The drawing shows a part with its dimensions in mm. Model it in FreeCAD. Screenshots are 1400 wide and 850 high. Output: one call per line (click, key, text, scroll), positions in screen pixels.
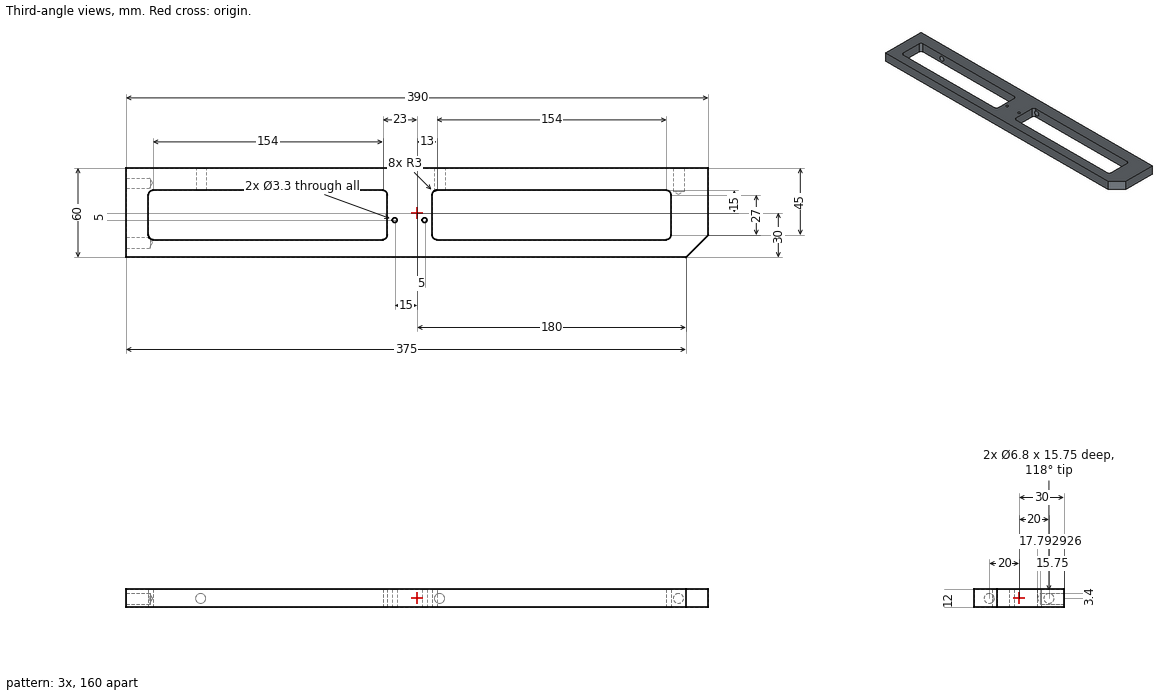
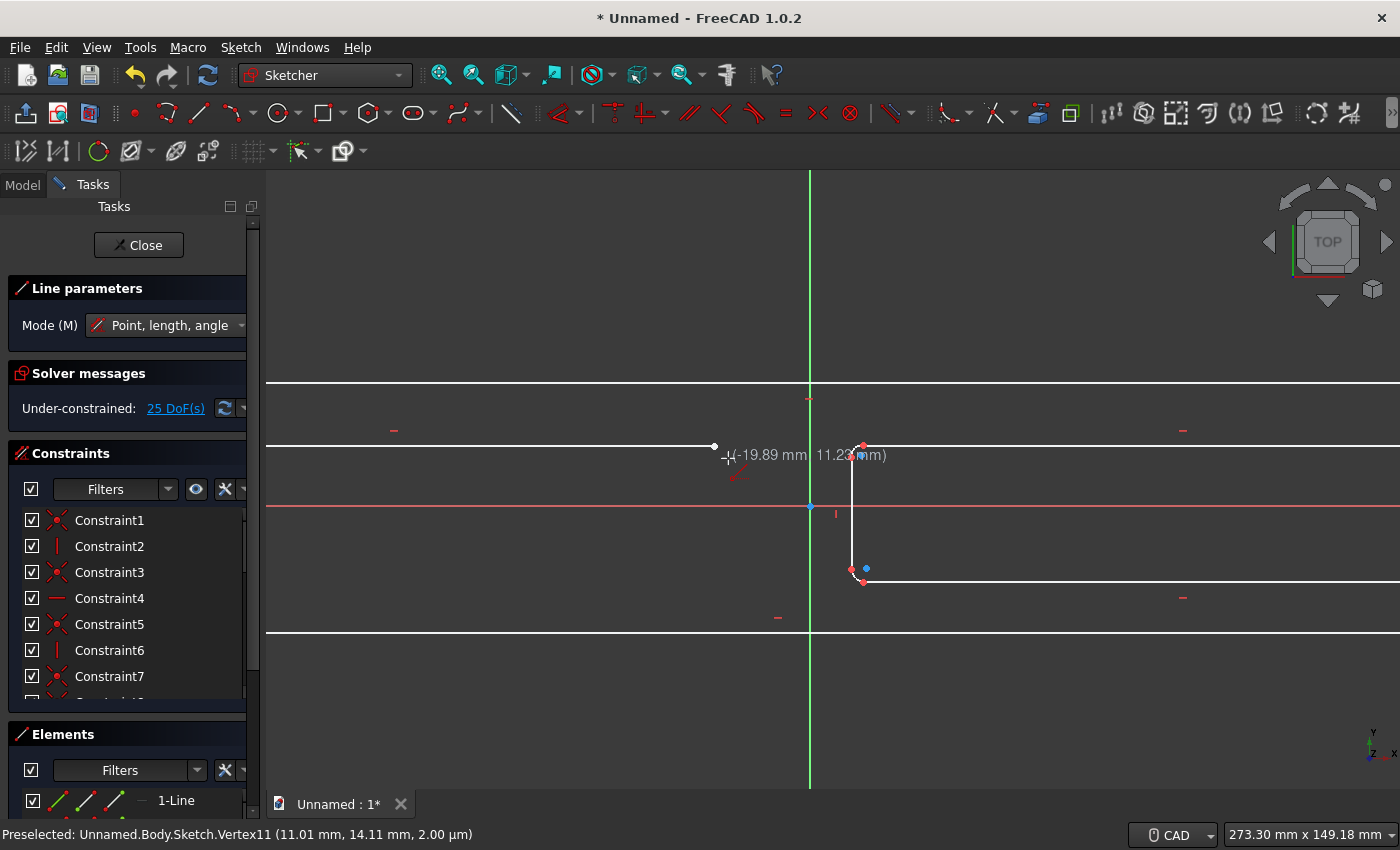
click(727, 456)
click(727, 568)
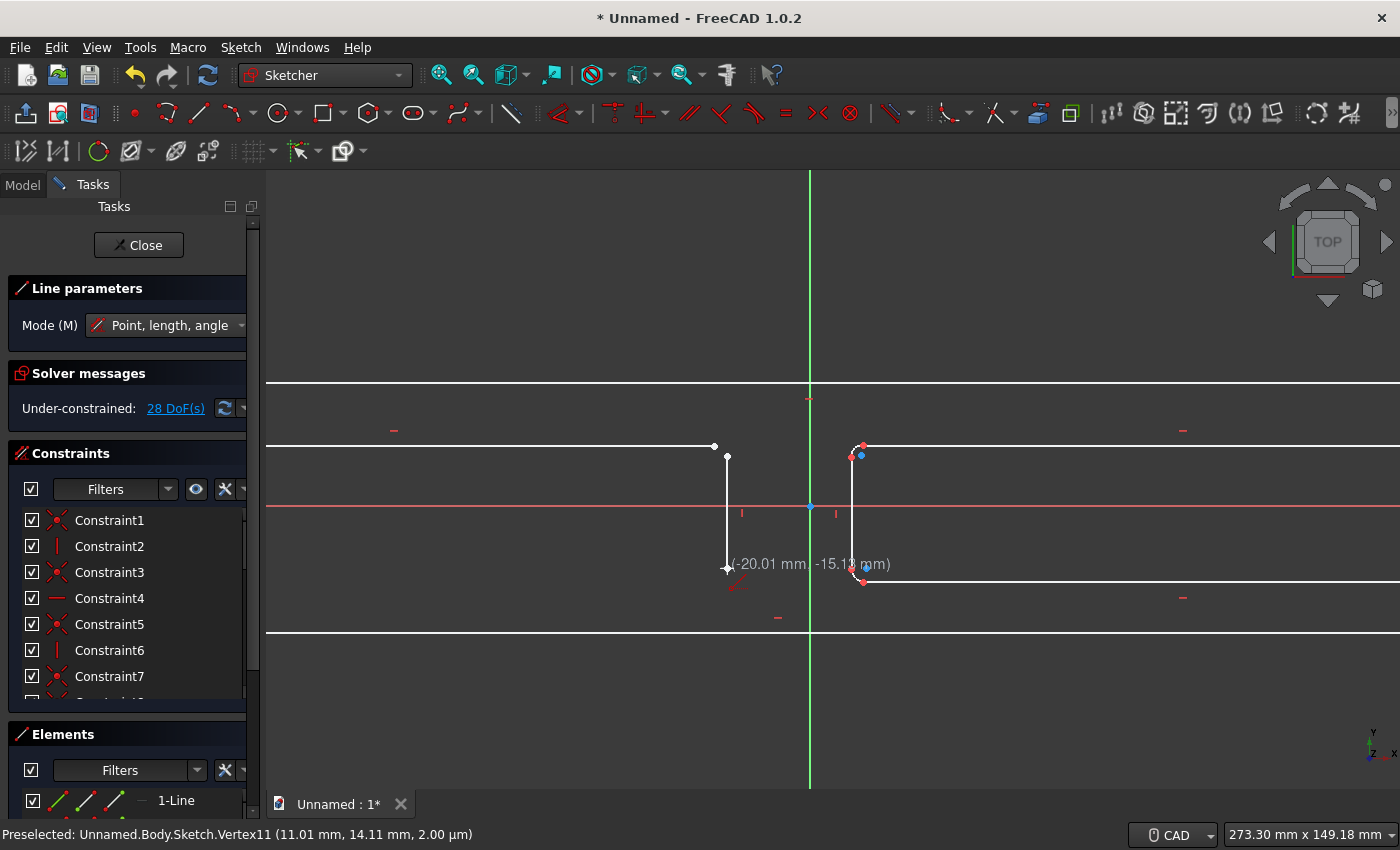
click(715, 581)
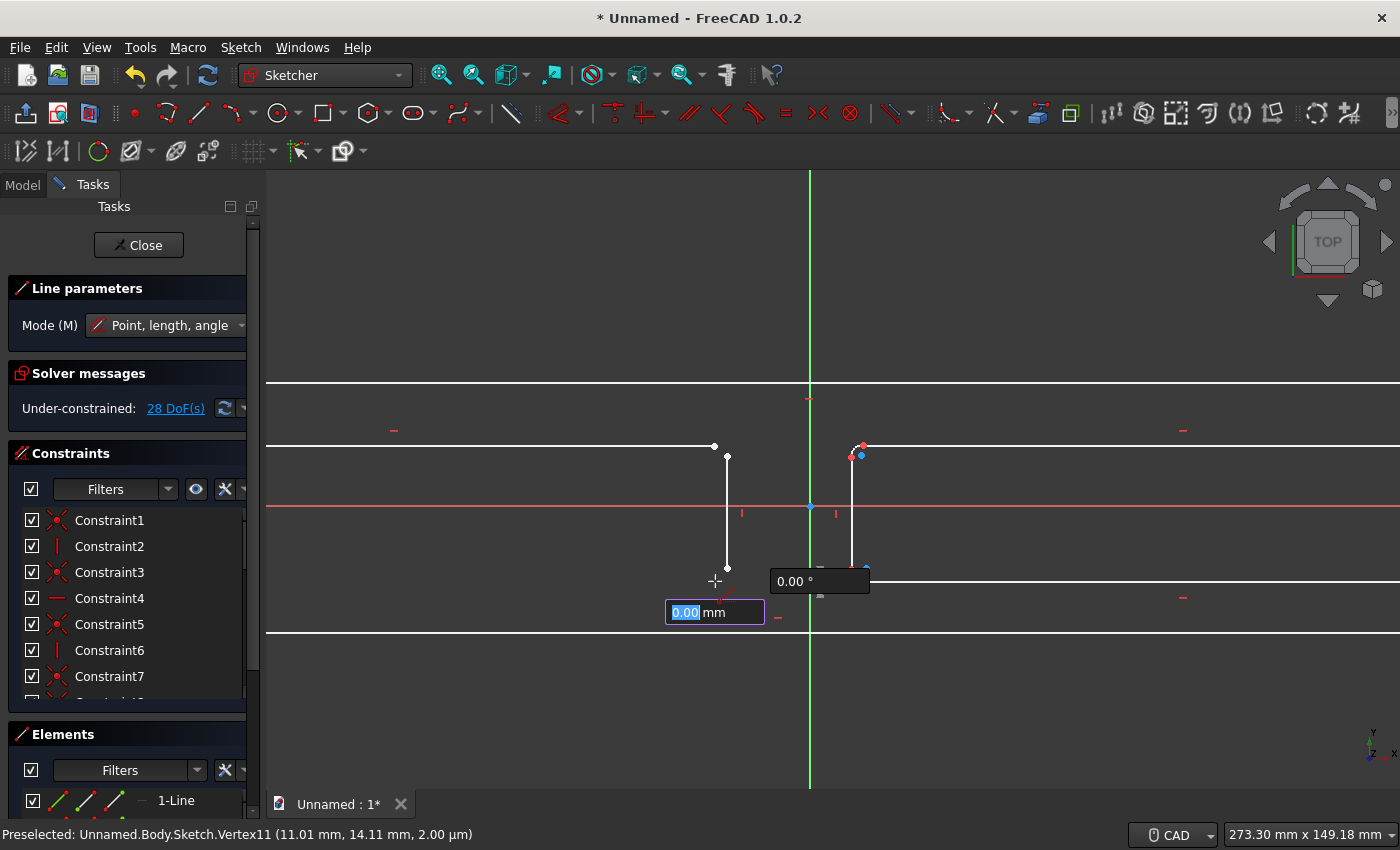
scroll(727, 458, down, 4)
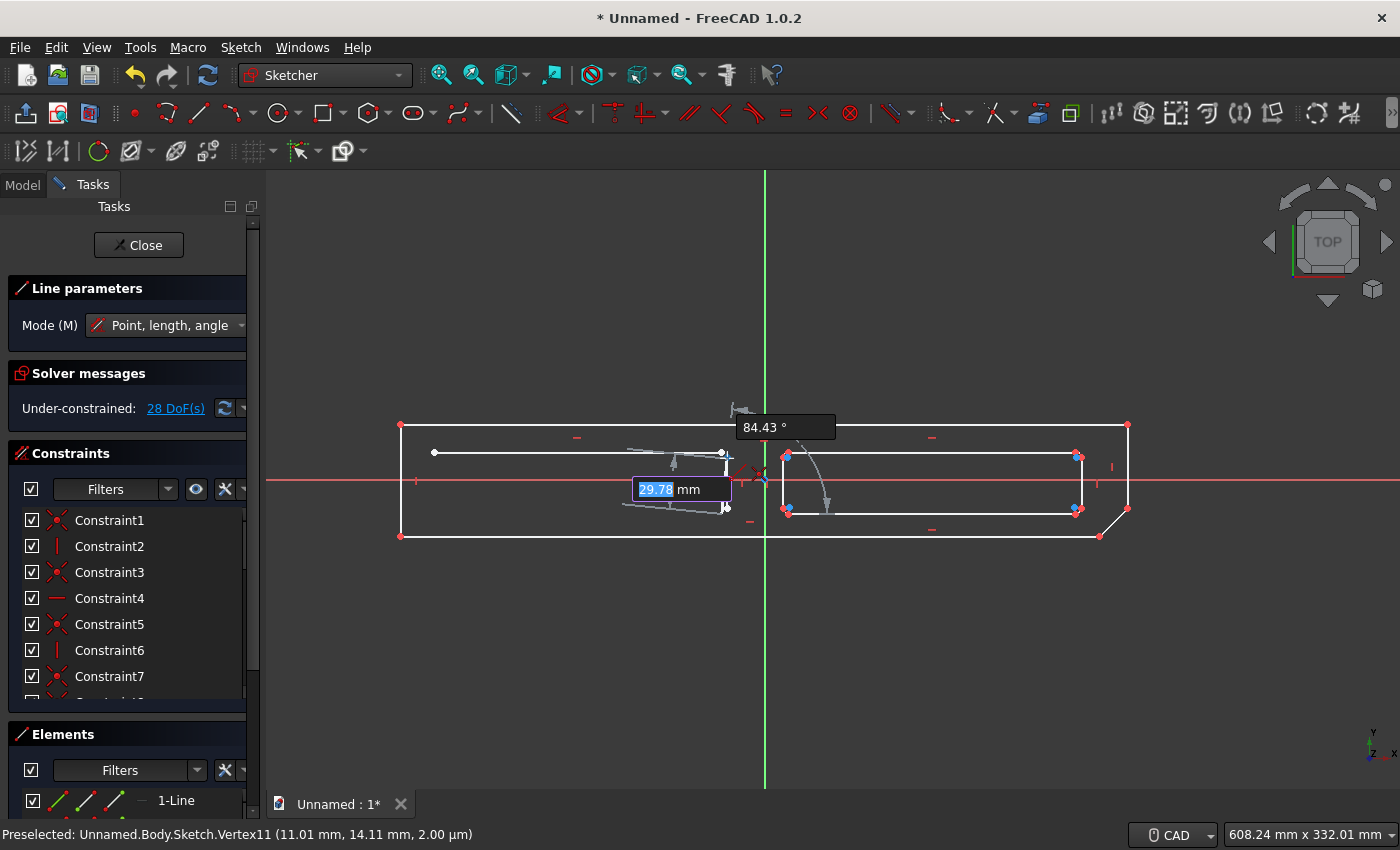
click(435, 514)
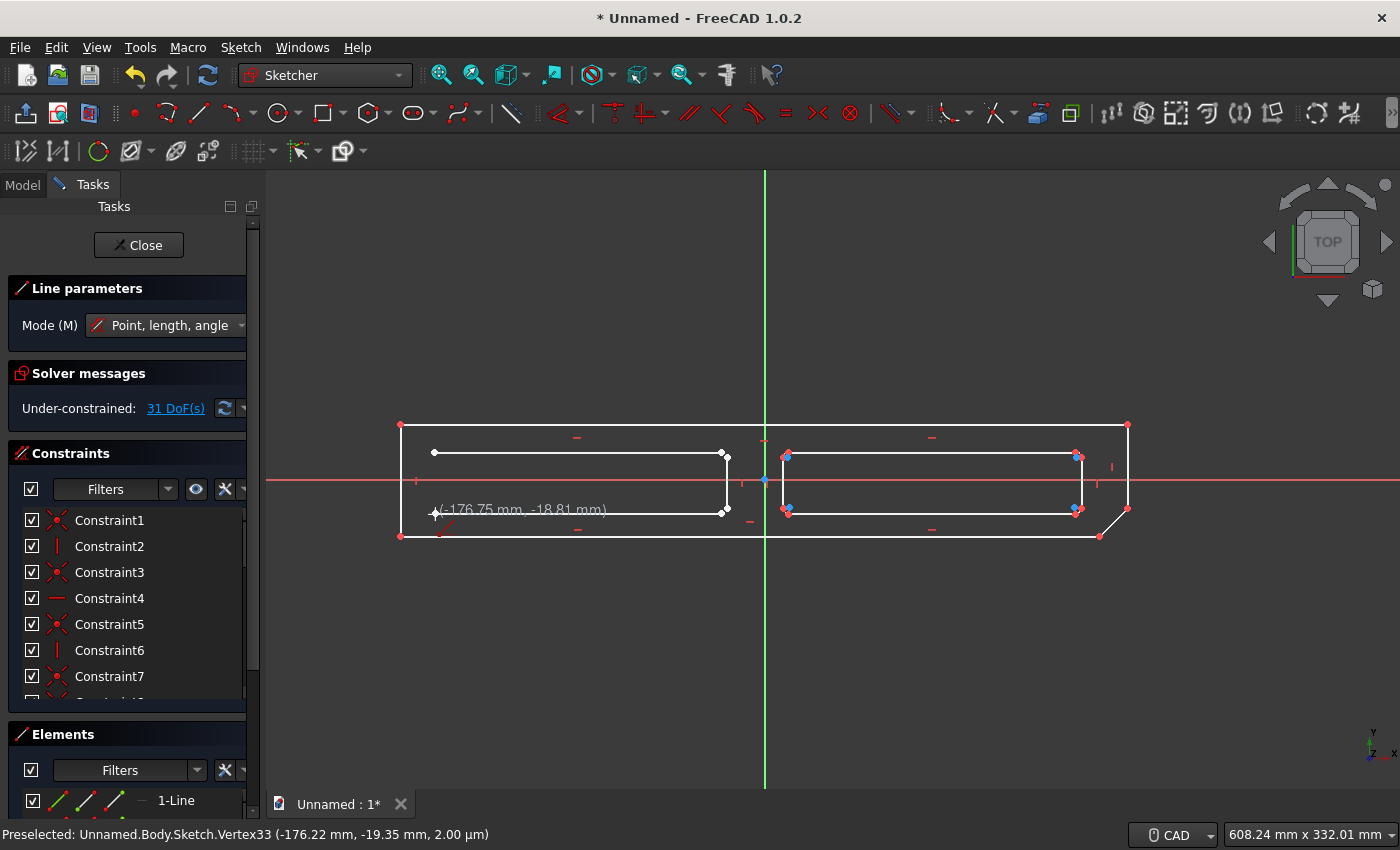
scroll(429, 508, up, 4)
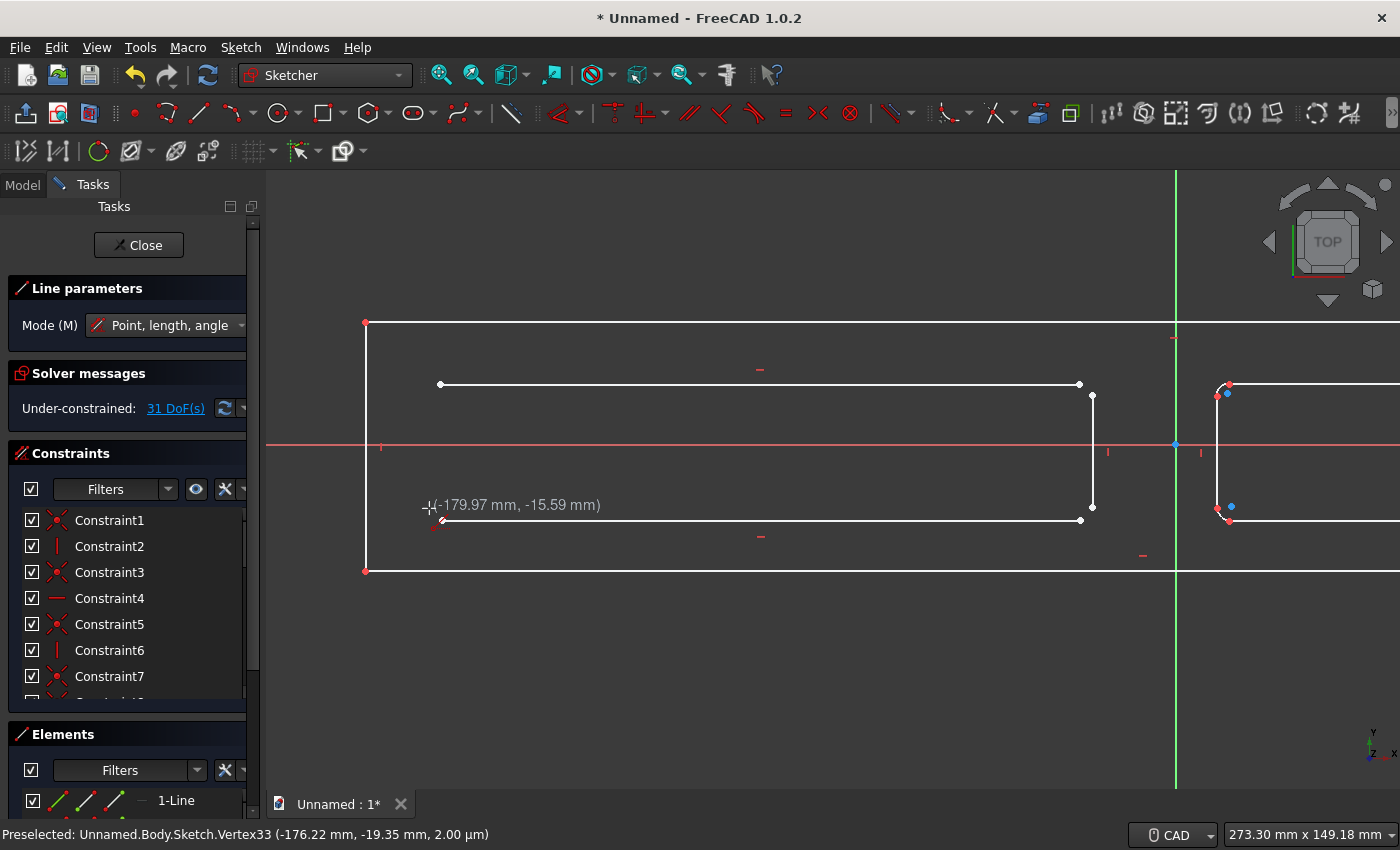
click(429, 507)
click(429, 395)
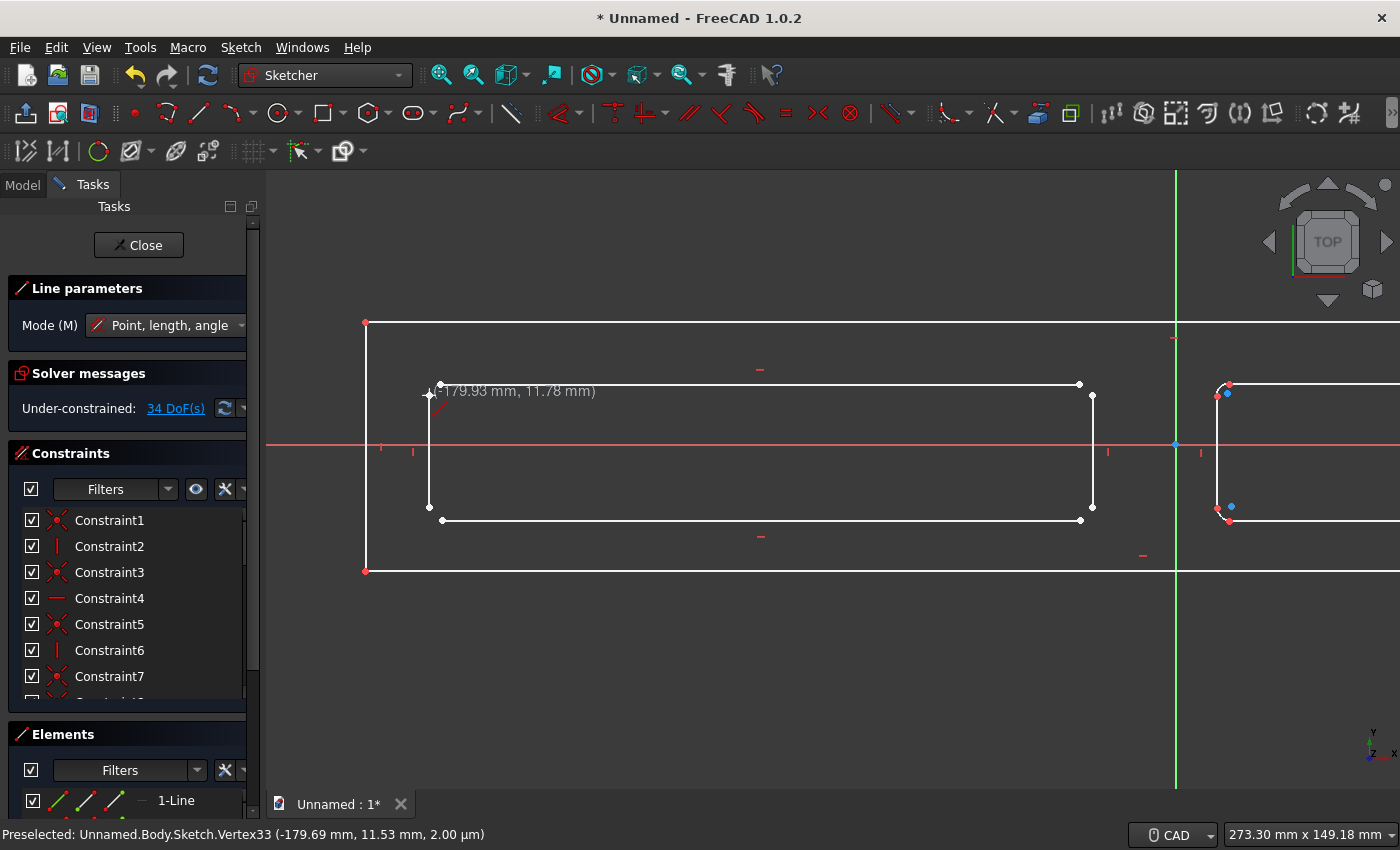
click(232, 114)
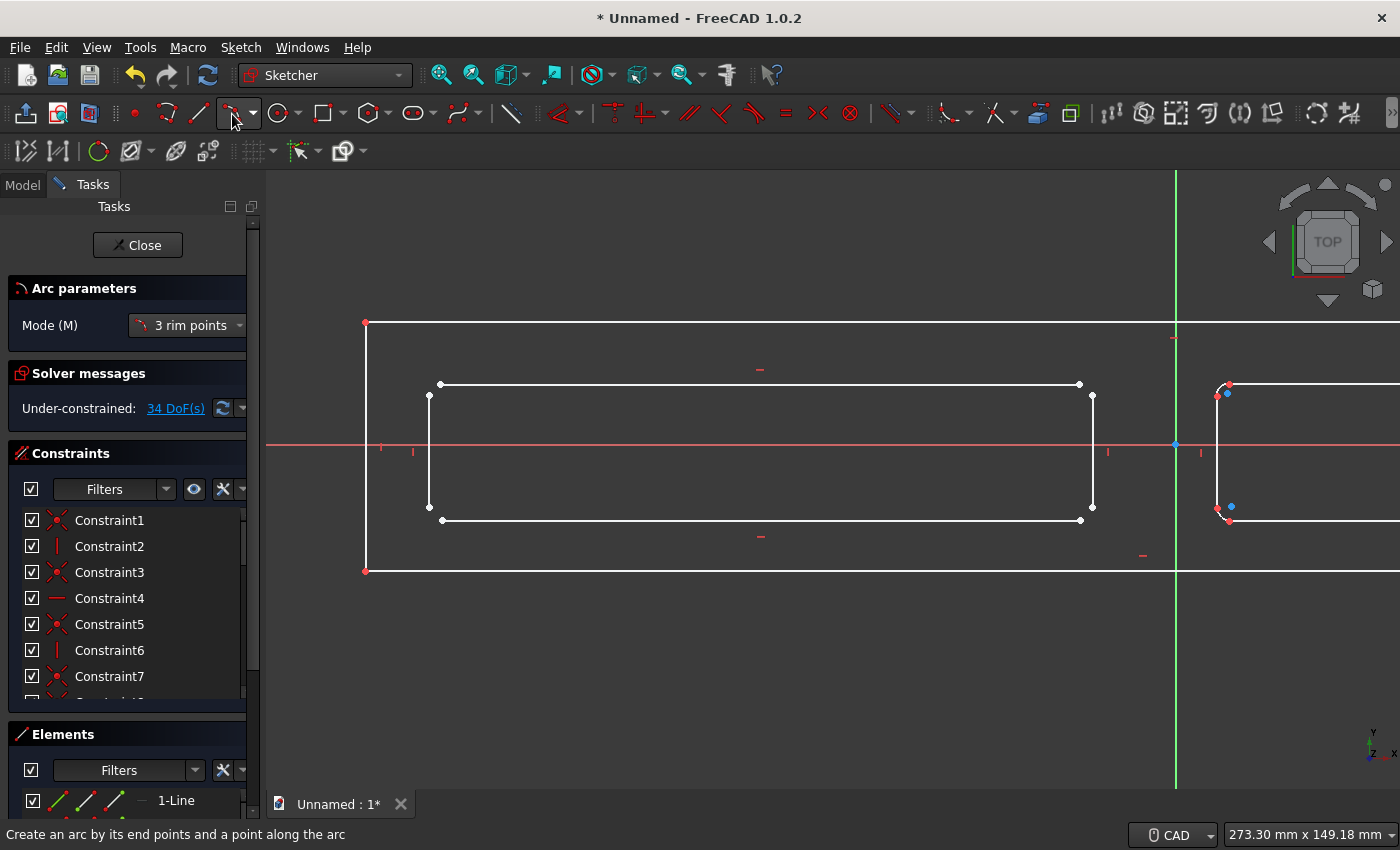
click(1080, 385)
click(1093, 396)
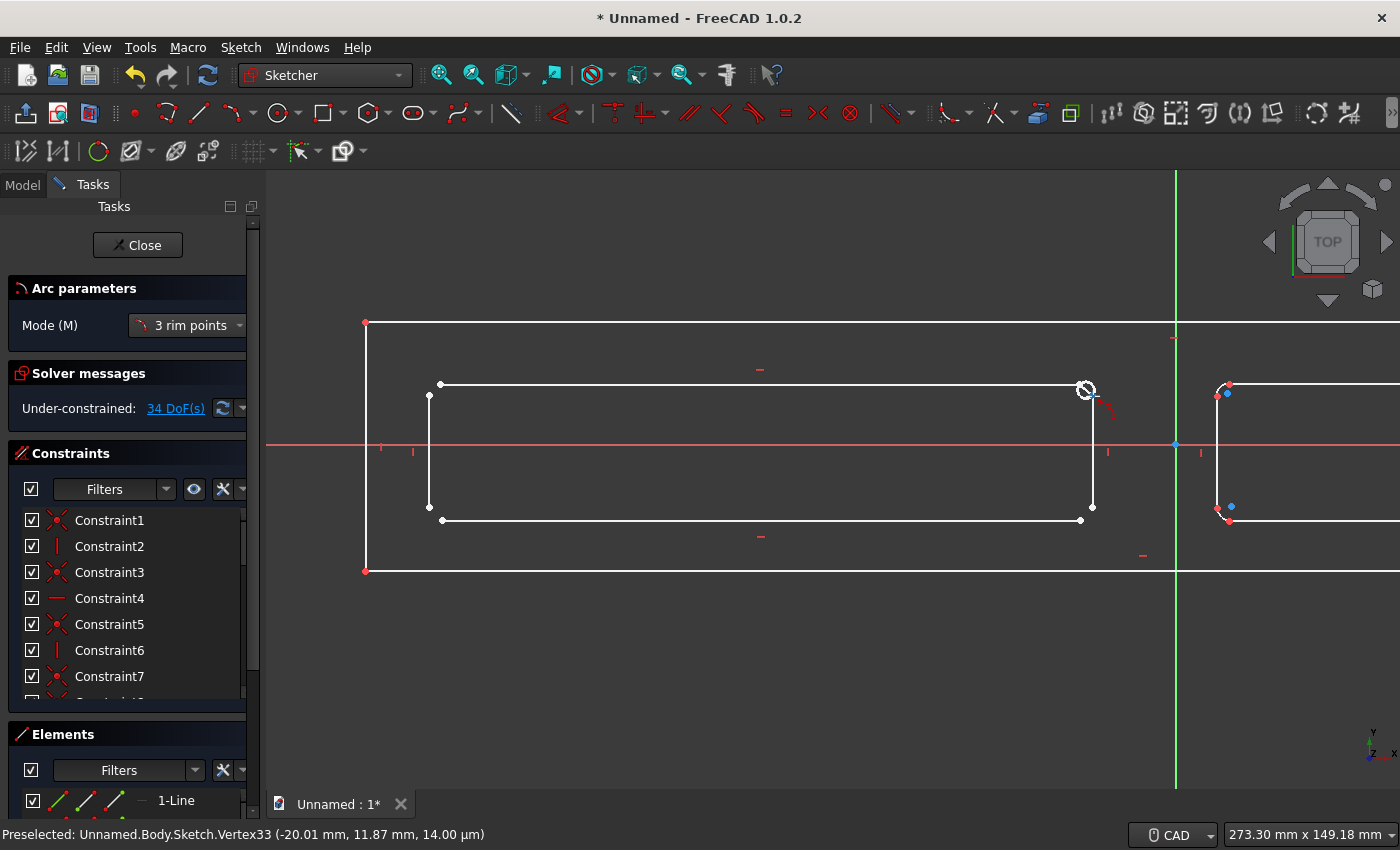
scroll(1089, 386, up, 8)